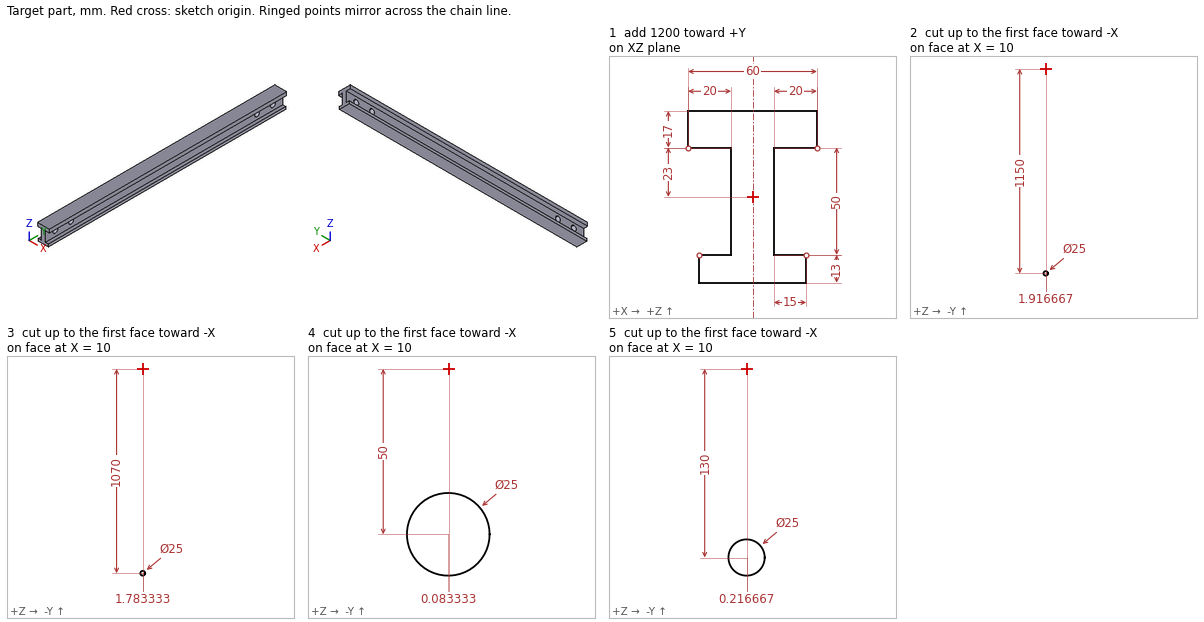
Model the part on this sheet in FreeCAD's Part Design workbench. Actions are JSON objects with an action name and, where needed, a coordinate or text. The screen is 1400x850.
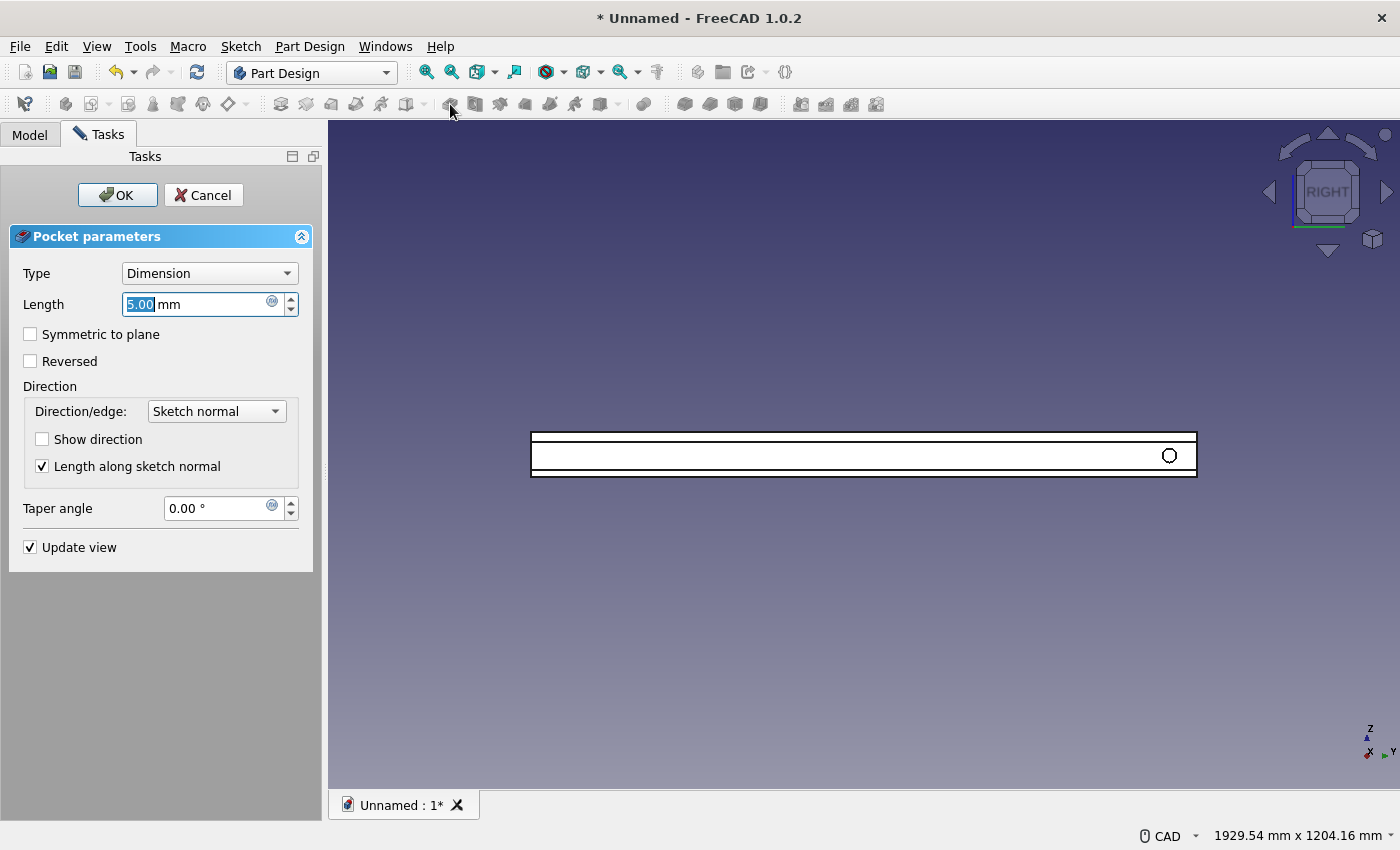
{"action": "left_click", "coordinate": [210, 274]}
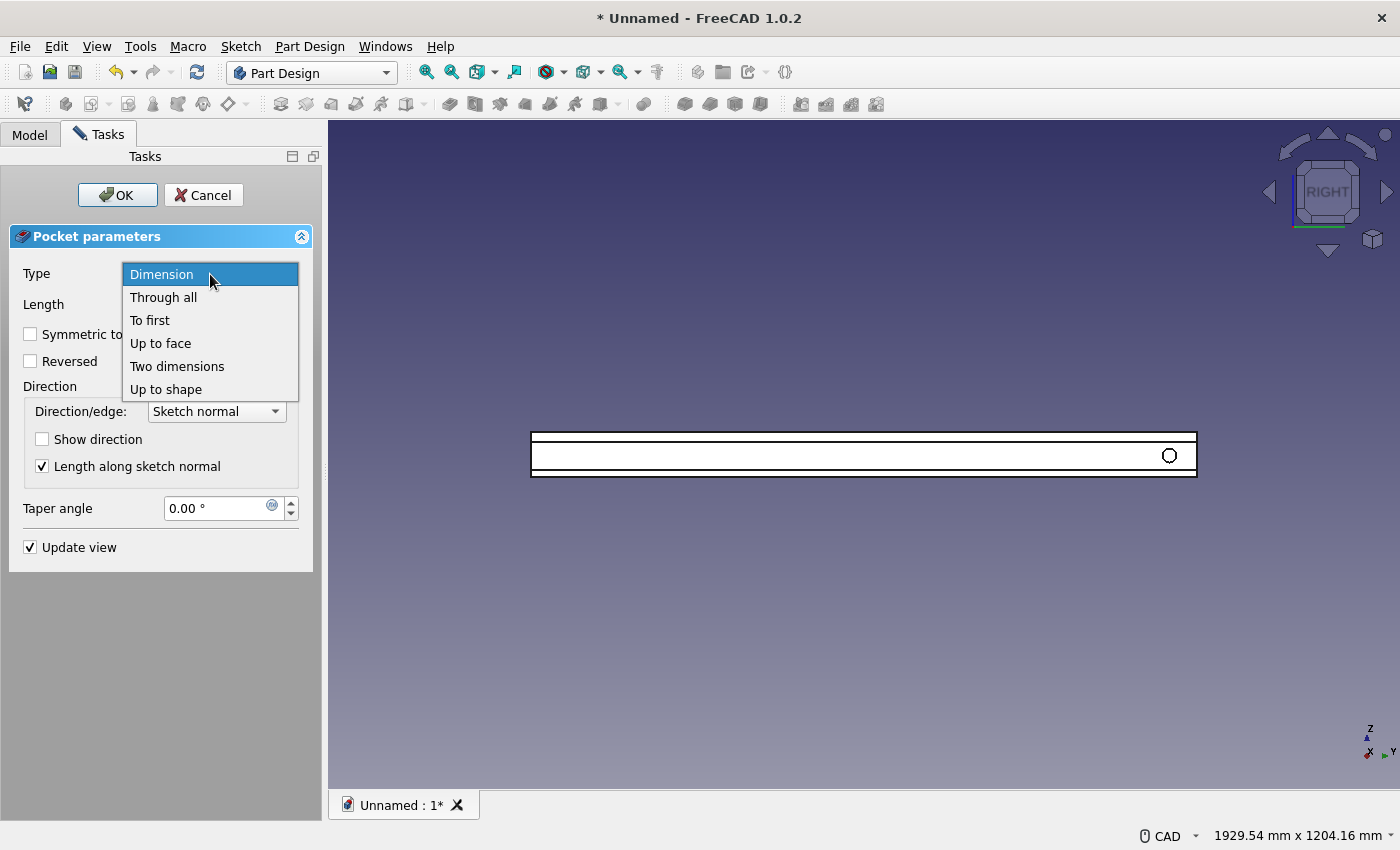
{"action": "left_click", "coordinate": [208, 320]}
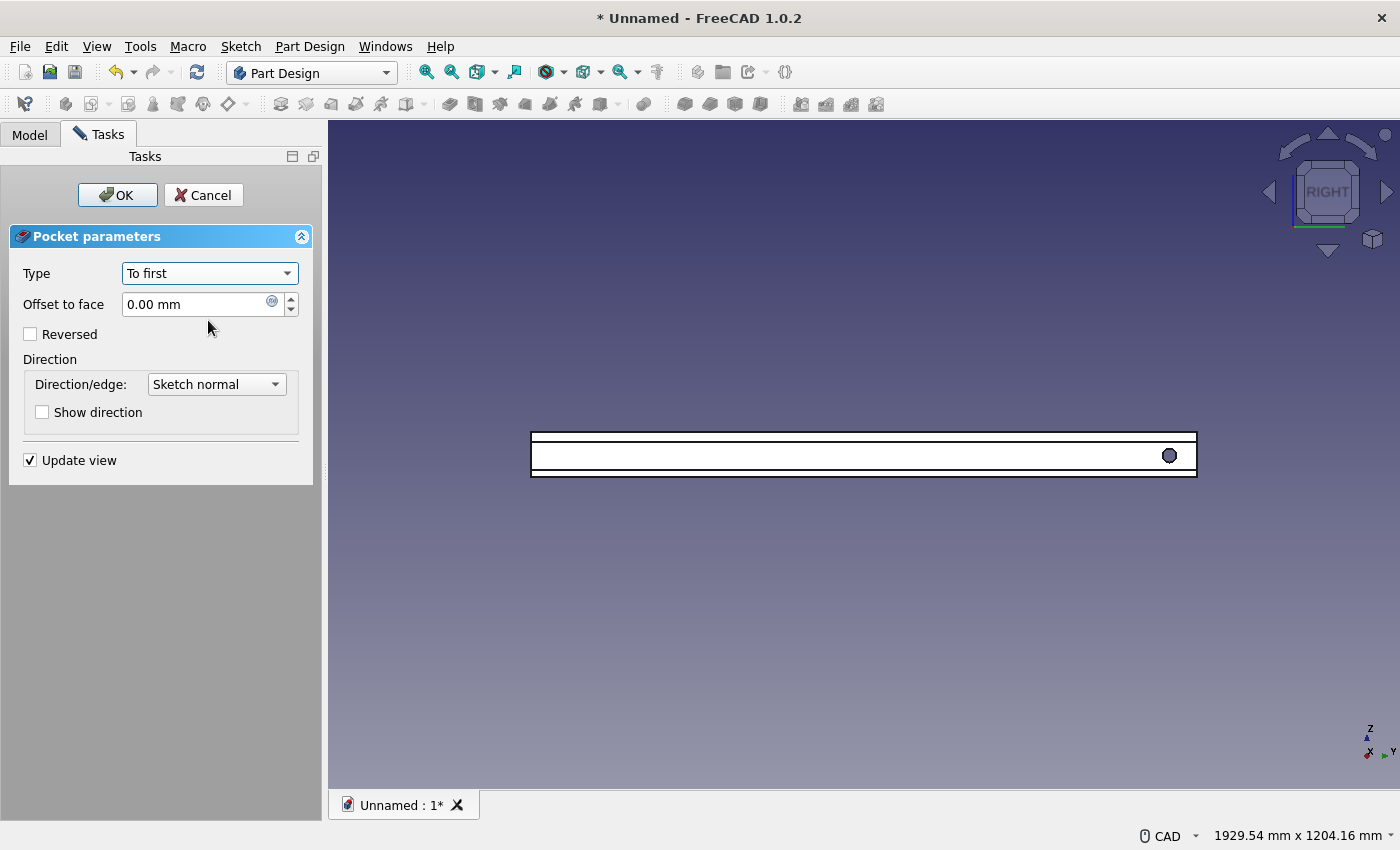
{"action": "left_click", "coordinate": [118, 195]}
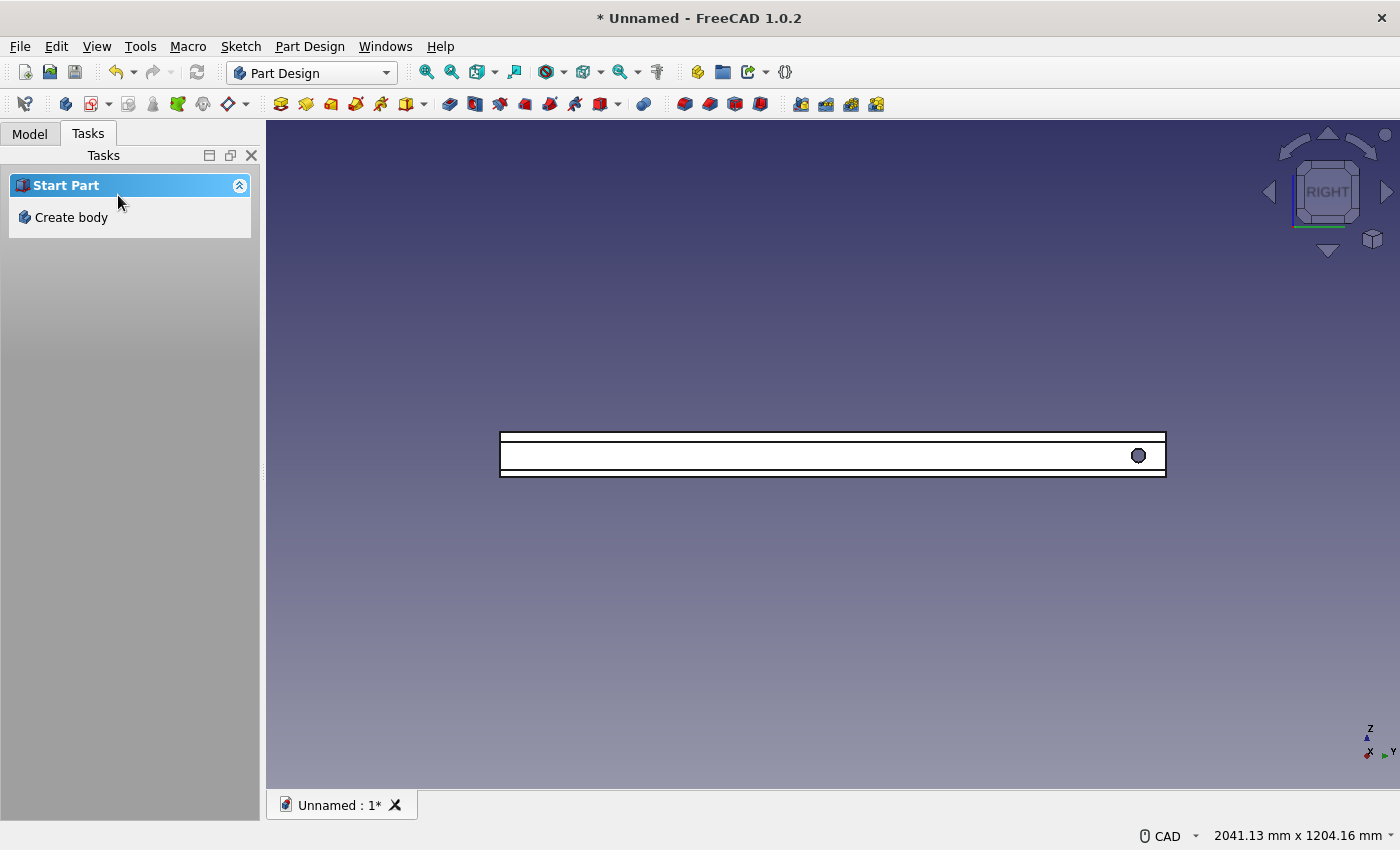
{"action": "left_click", "coordinate": [1023, 455]}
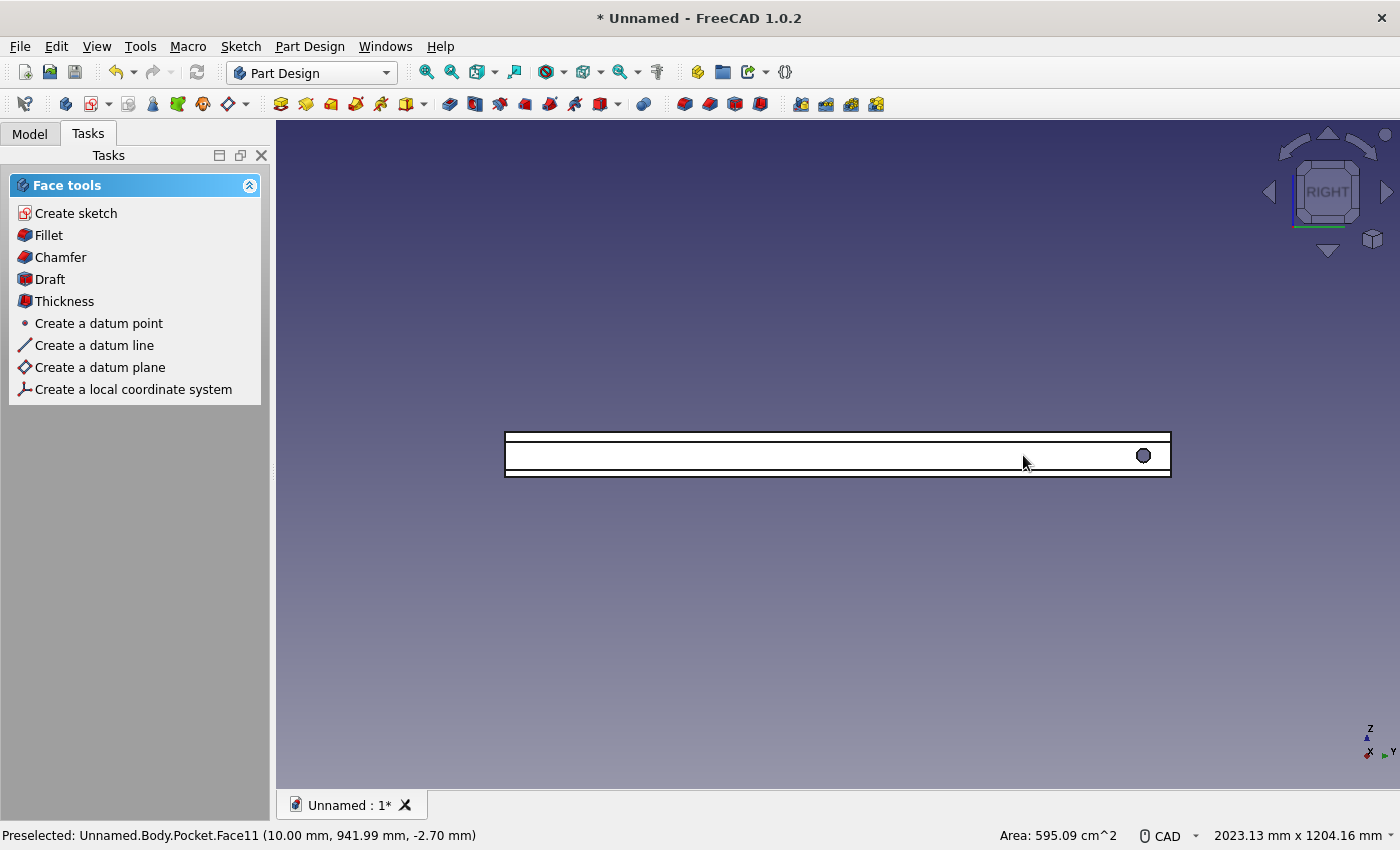
{"action": "left_click", "coordinate": [90, 104]}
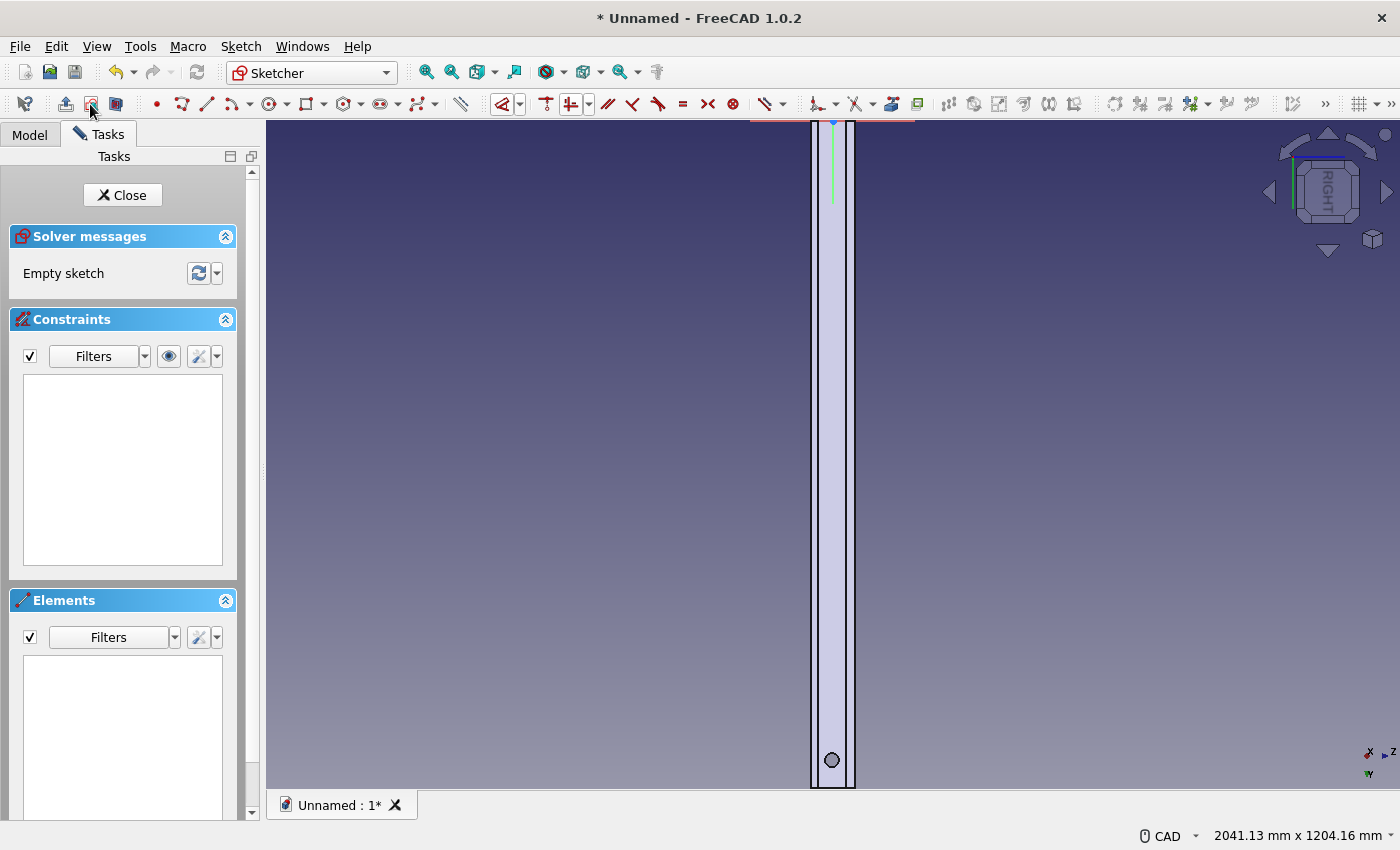
{"action": "scroll", "coordinate": [836, 729], "scroll_direction": "up", "scroll_amount": 15}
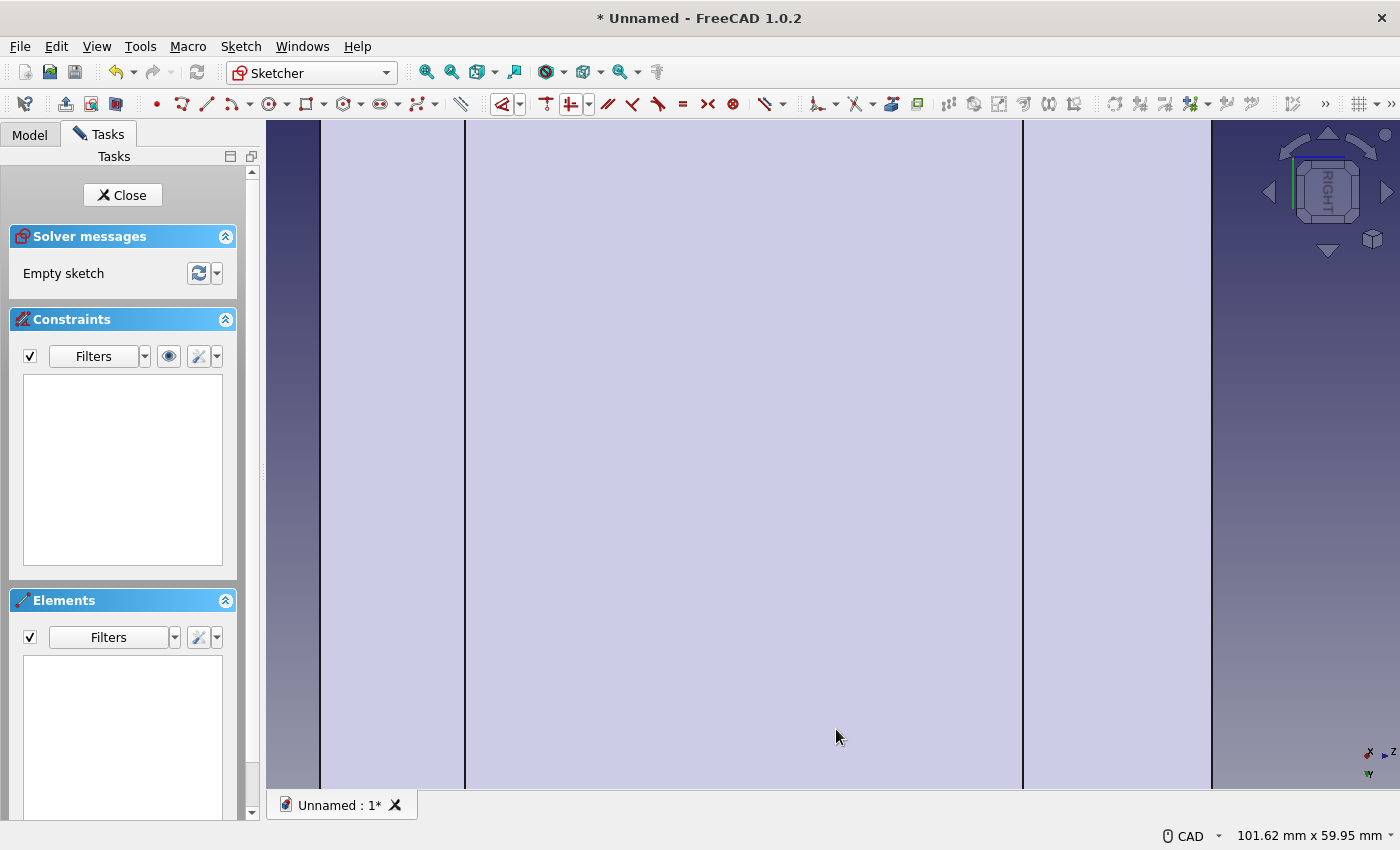
{"action": "scroll", "coordinate": [709, 419], "scroll_direction": "up", "scroll_amount": 2}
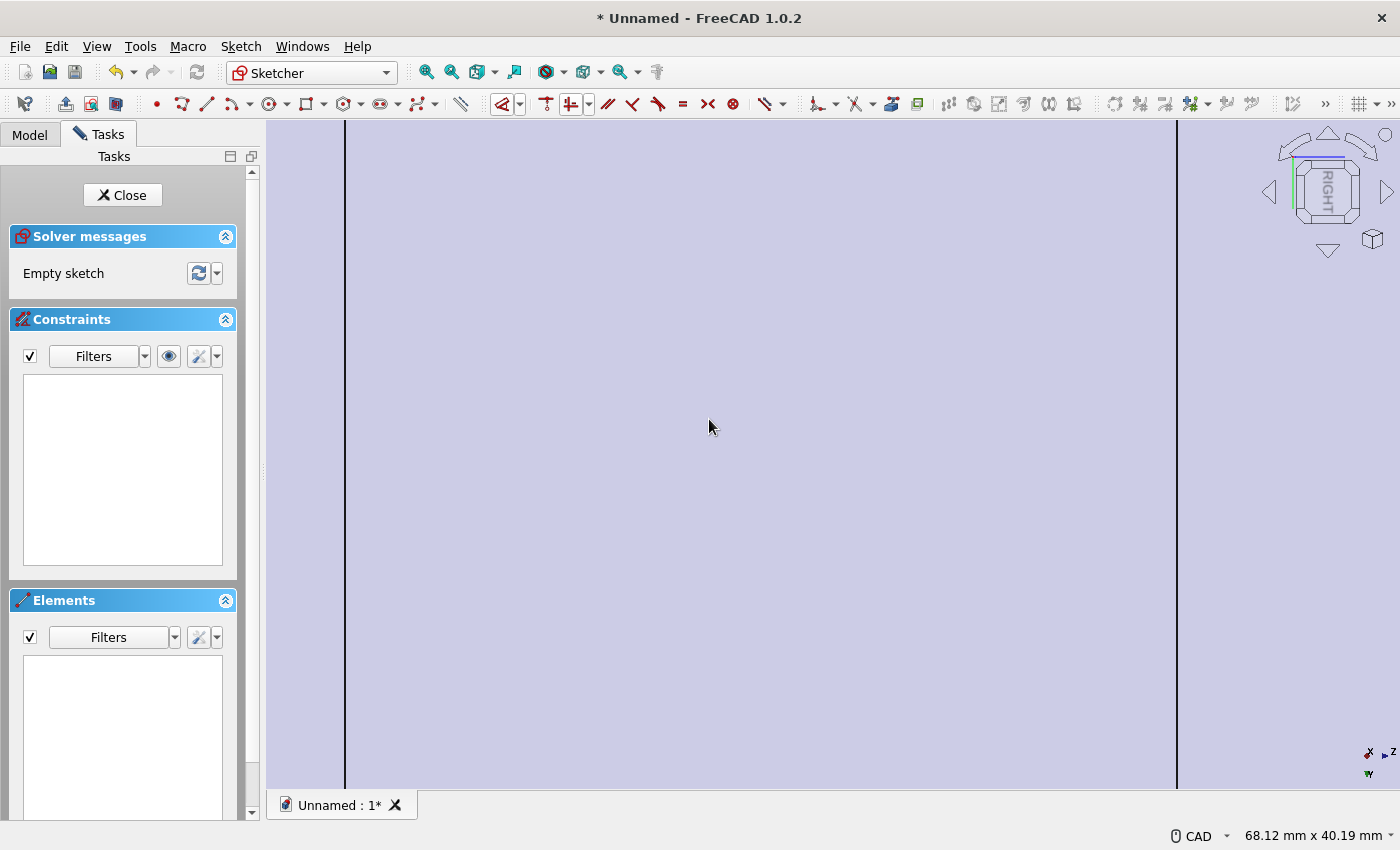
{"action": "left_click", "coordinate": [268, 104]}